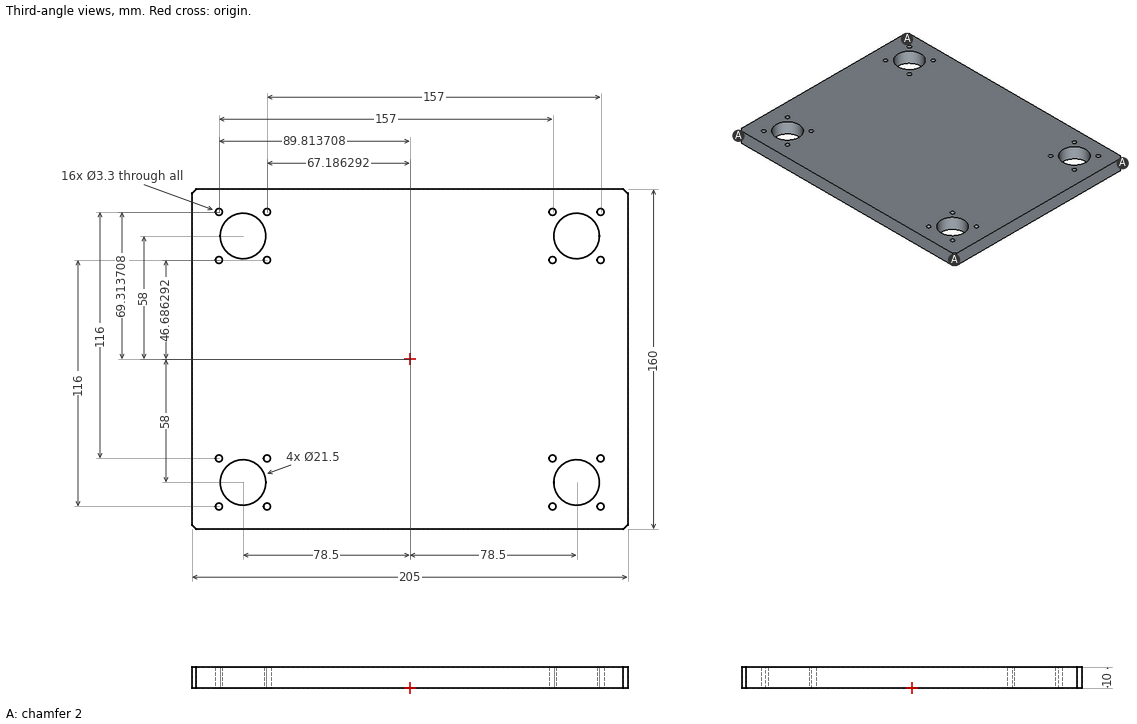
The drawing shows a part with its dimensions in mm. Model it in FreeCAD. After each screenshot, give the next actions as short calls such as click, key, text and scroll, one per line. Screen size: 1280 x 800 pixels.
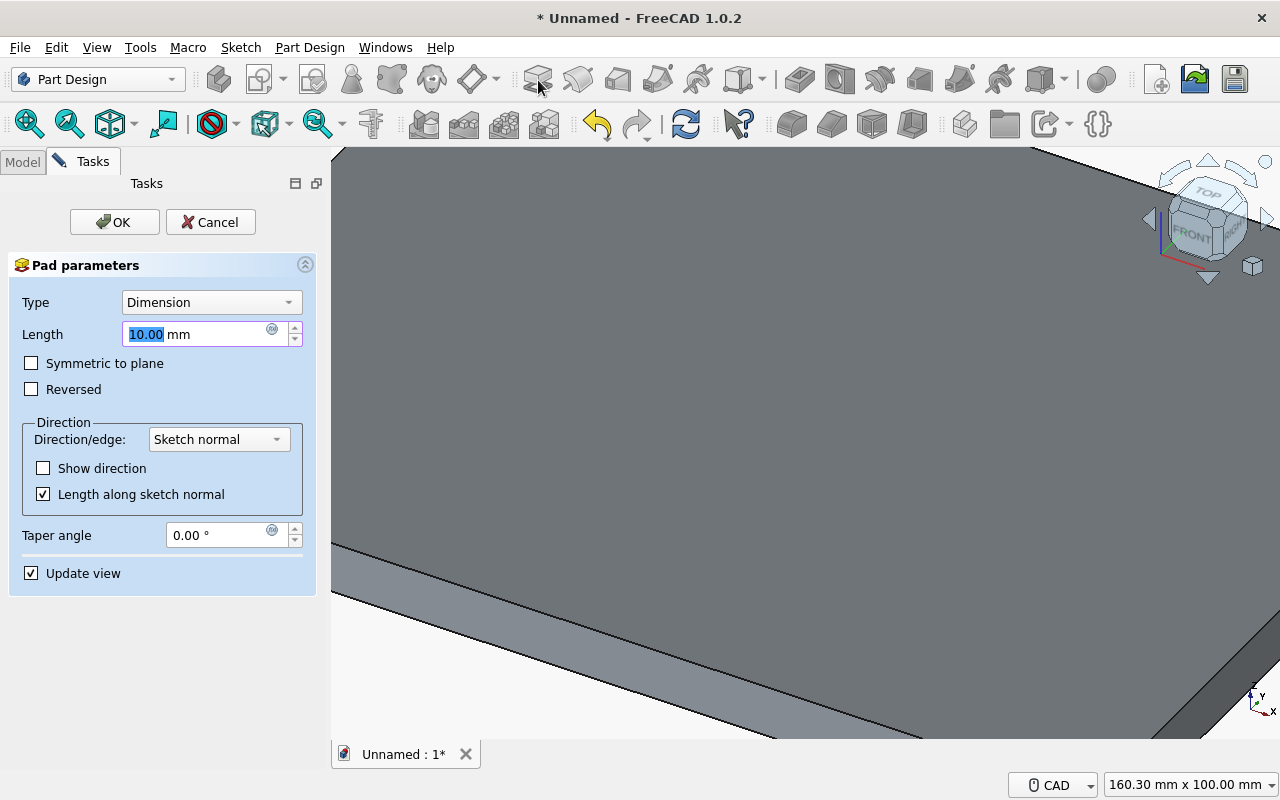
text(10)
key(Tab)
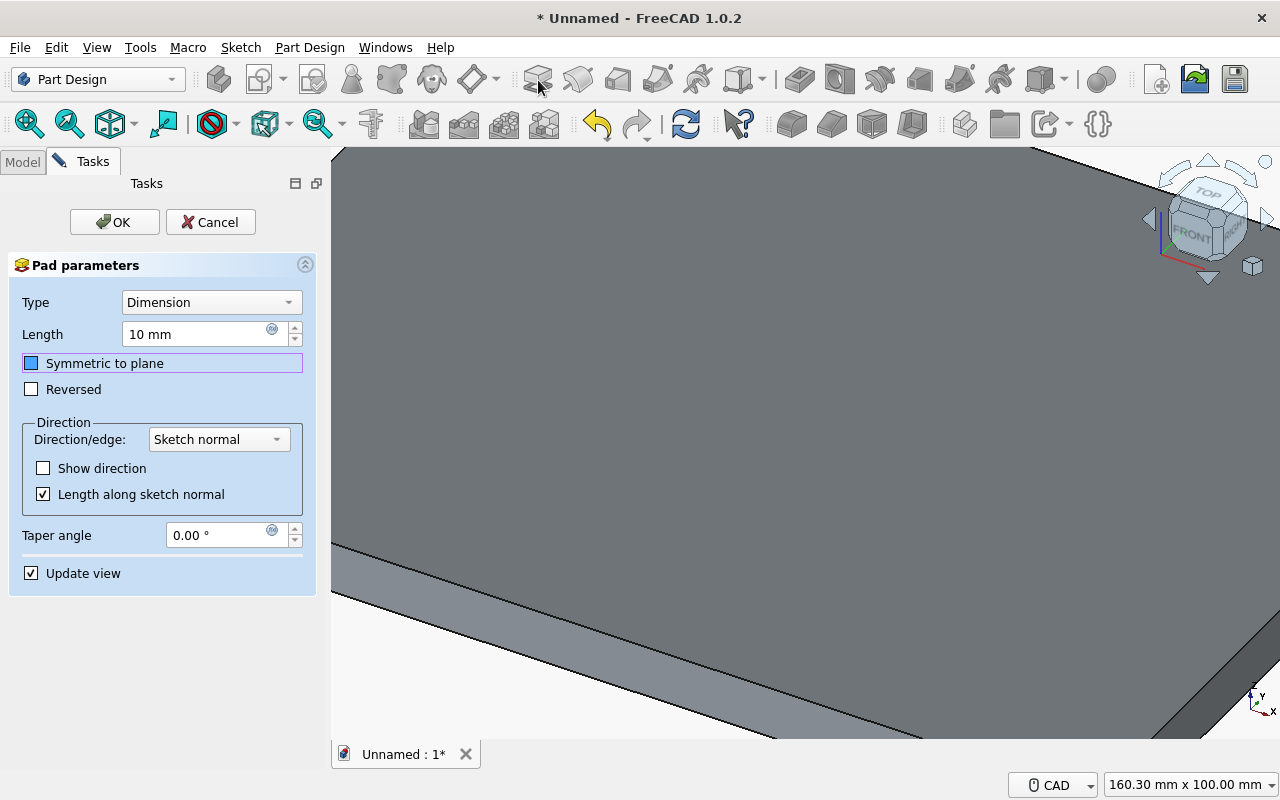
click(115, 222)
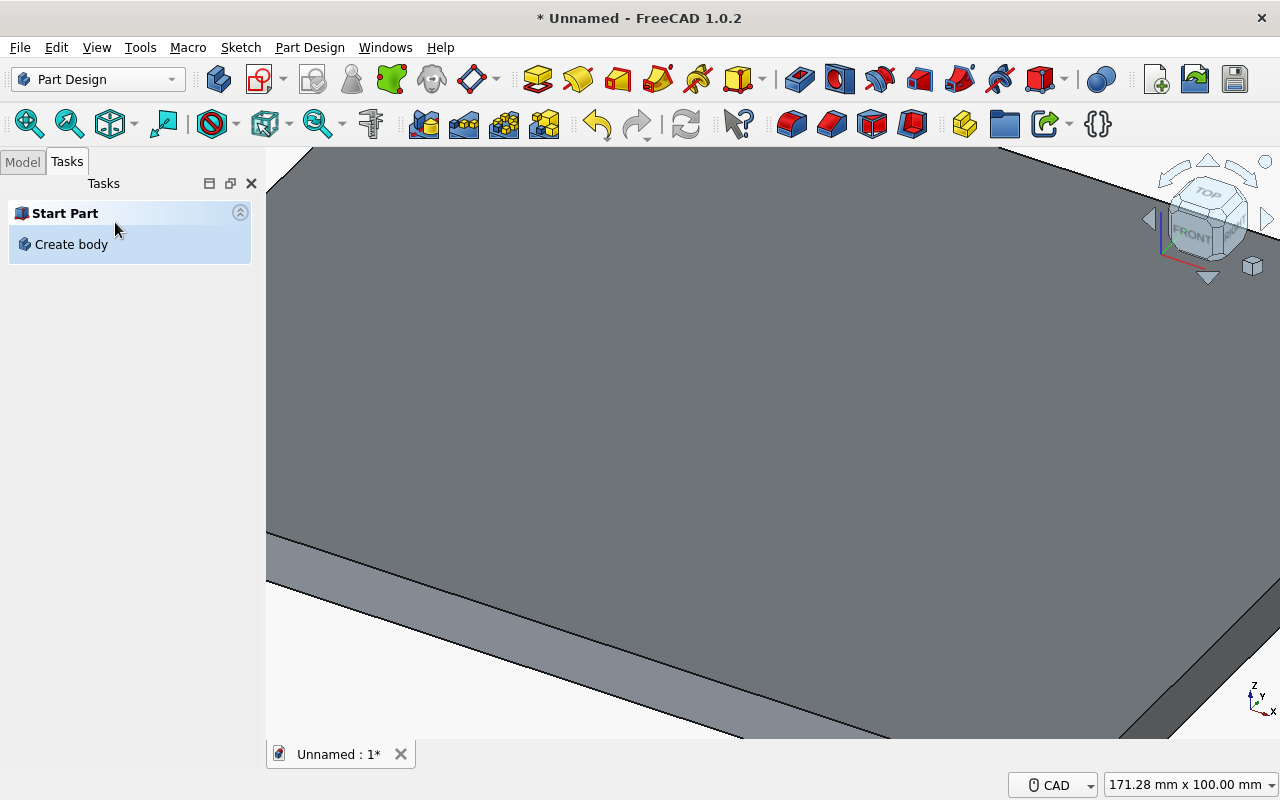
key(v)
key(f)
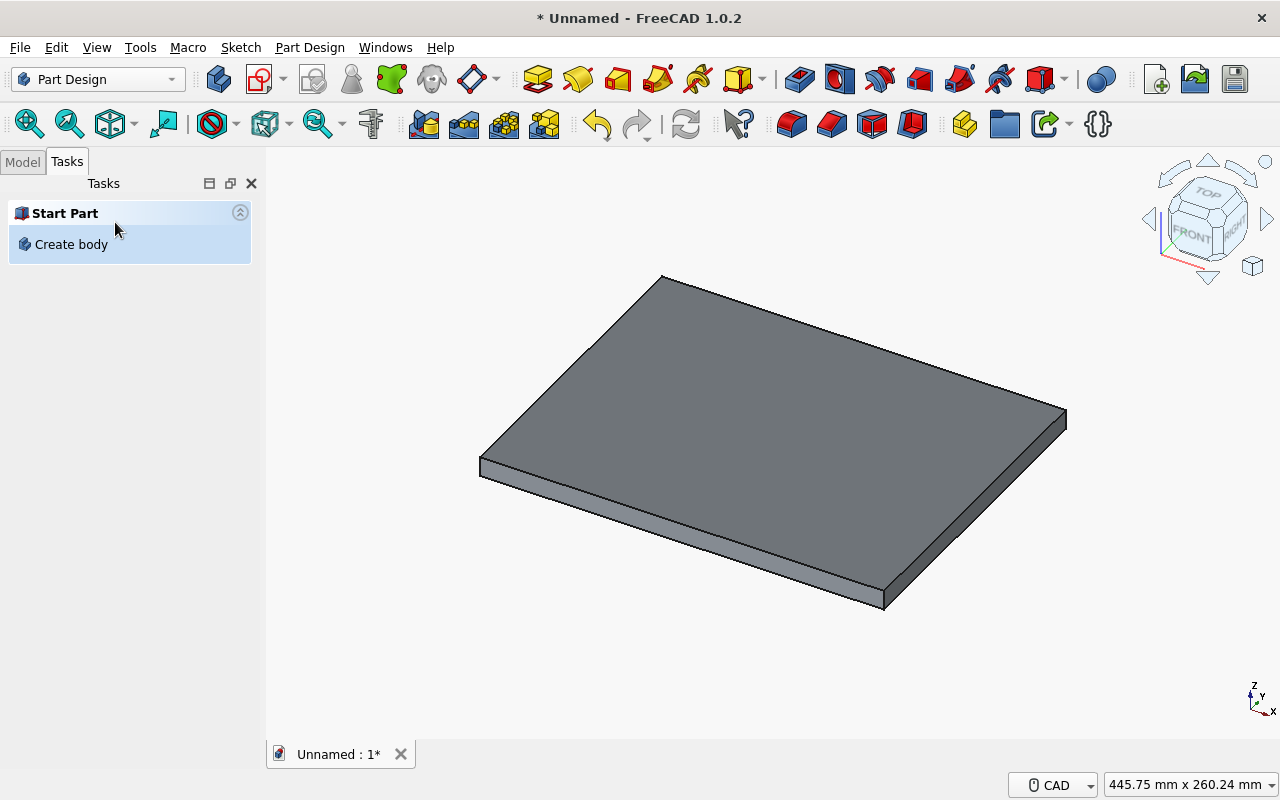
click(773, 433)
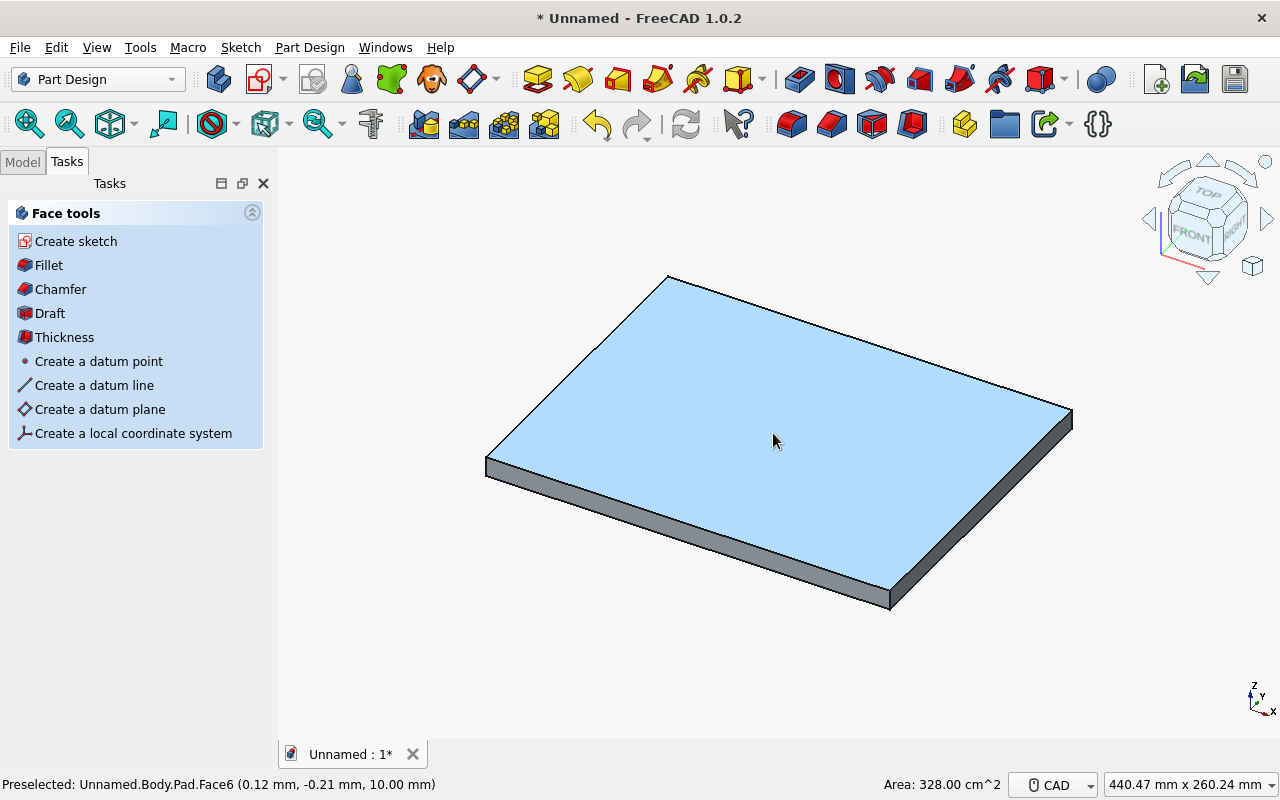
click(260, 80)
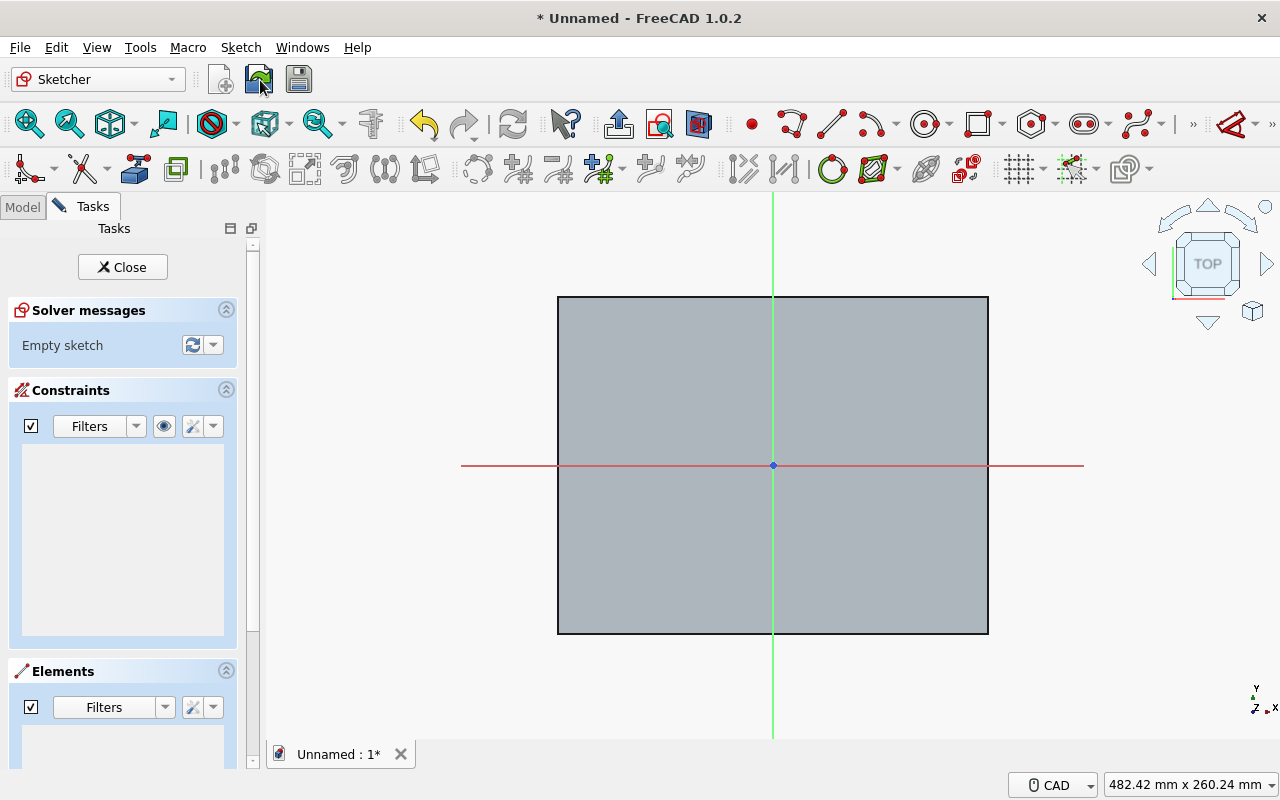
key(g)
key(c)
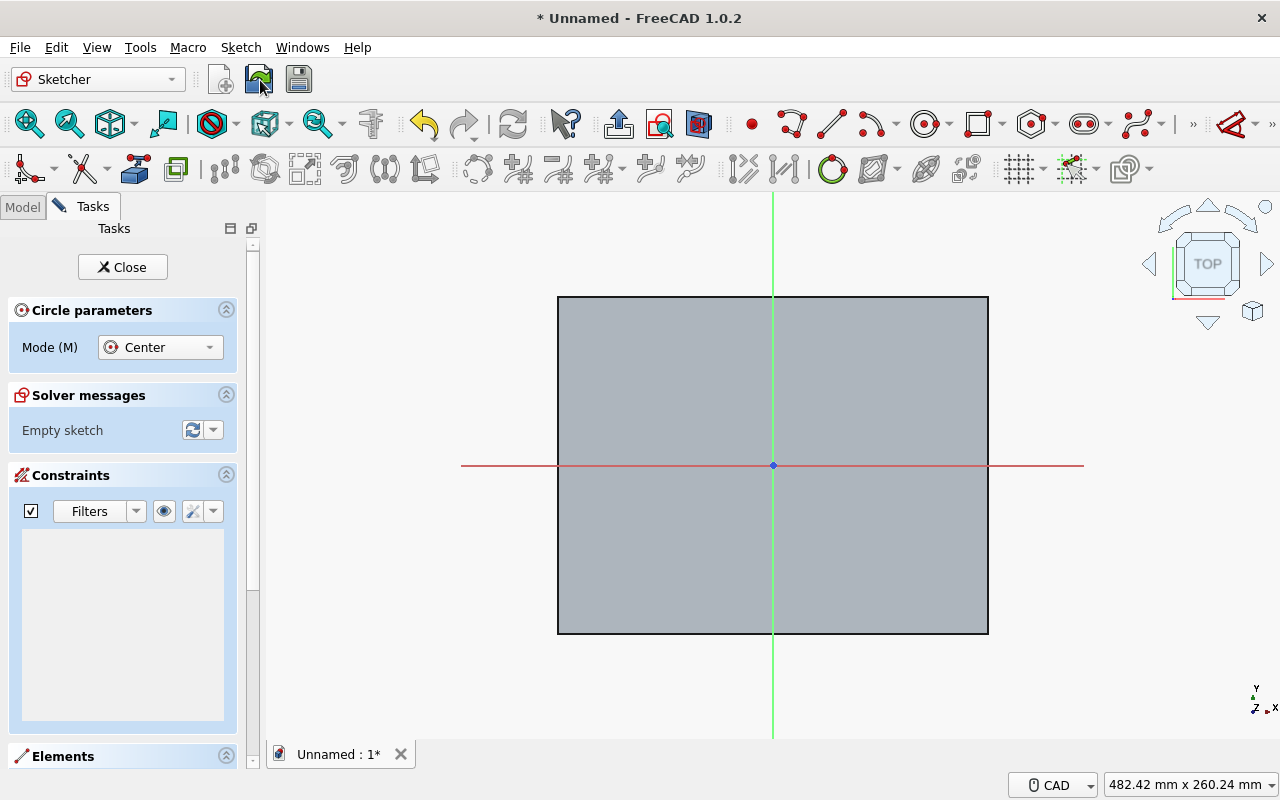
click(608, 587)
move(624, 571)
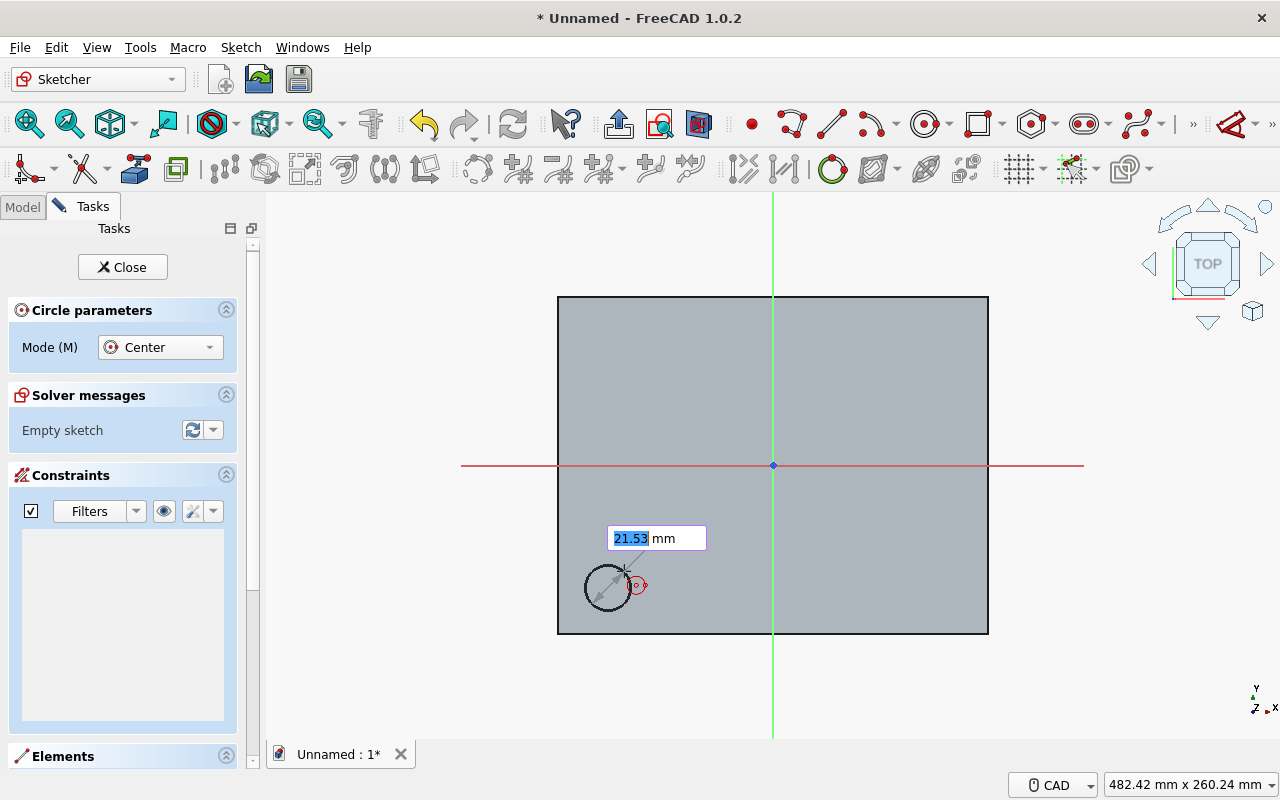
text(21.5)
key(Return)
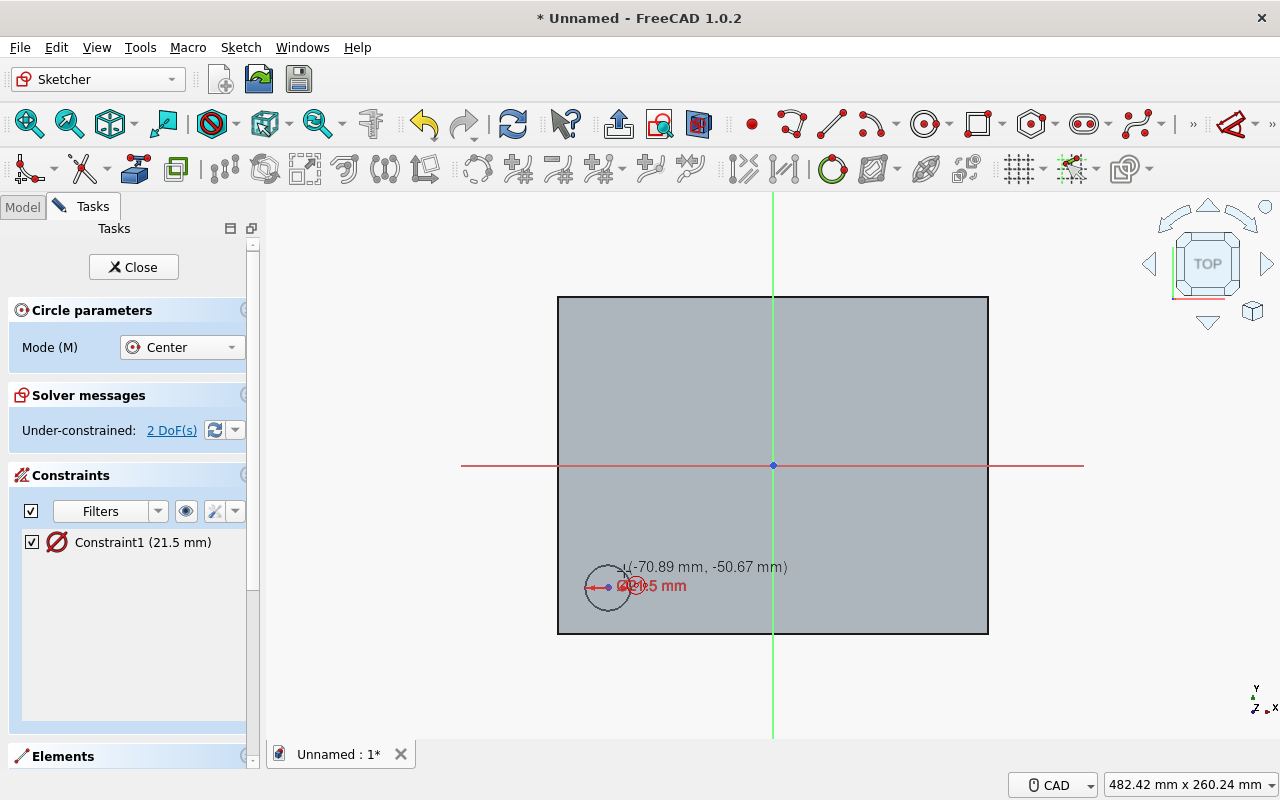
click(608, 344)
move(624, 328)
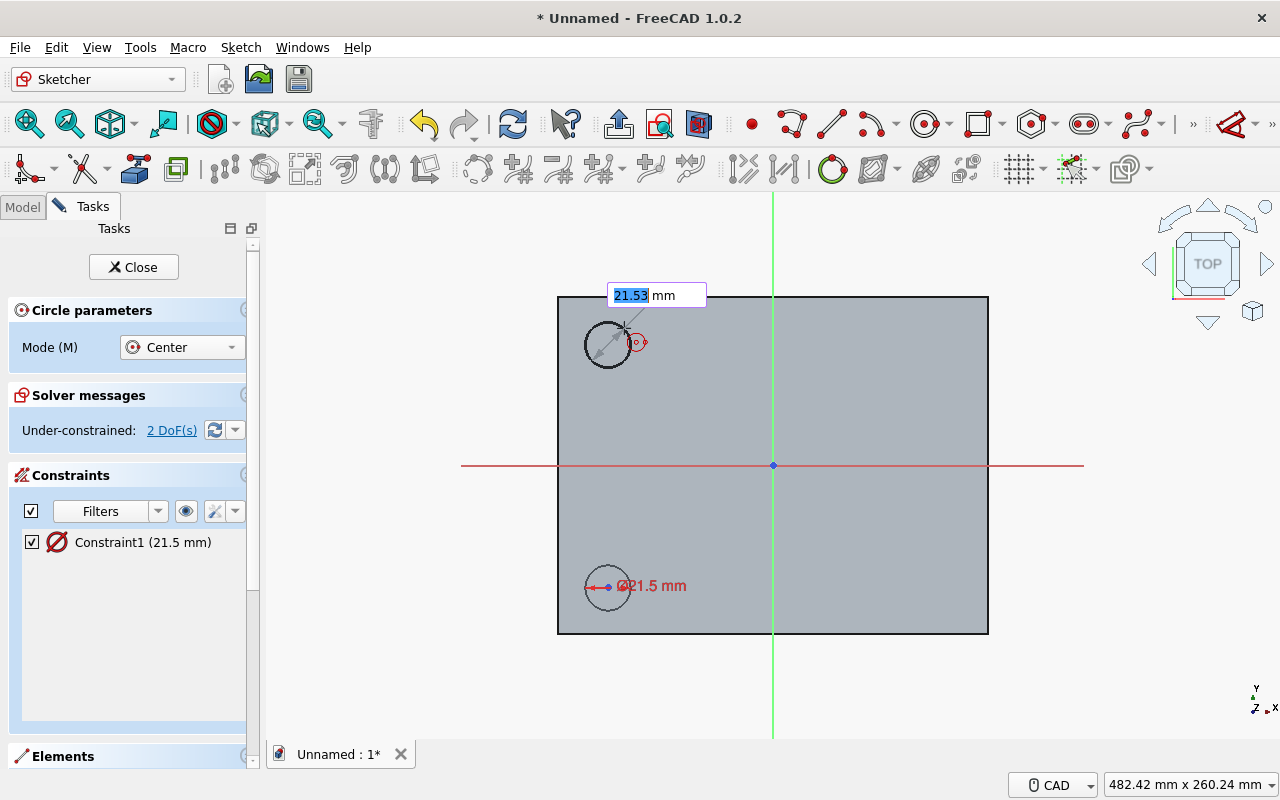
text(21.5)
key(Return)